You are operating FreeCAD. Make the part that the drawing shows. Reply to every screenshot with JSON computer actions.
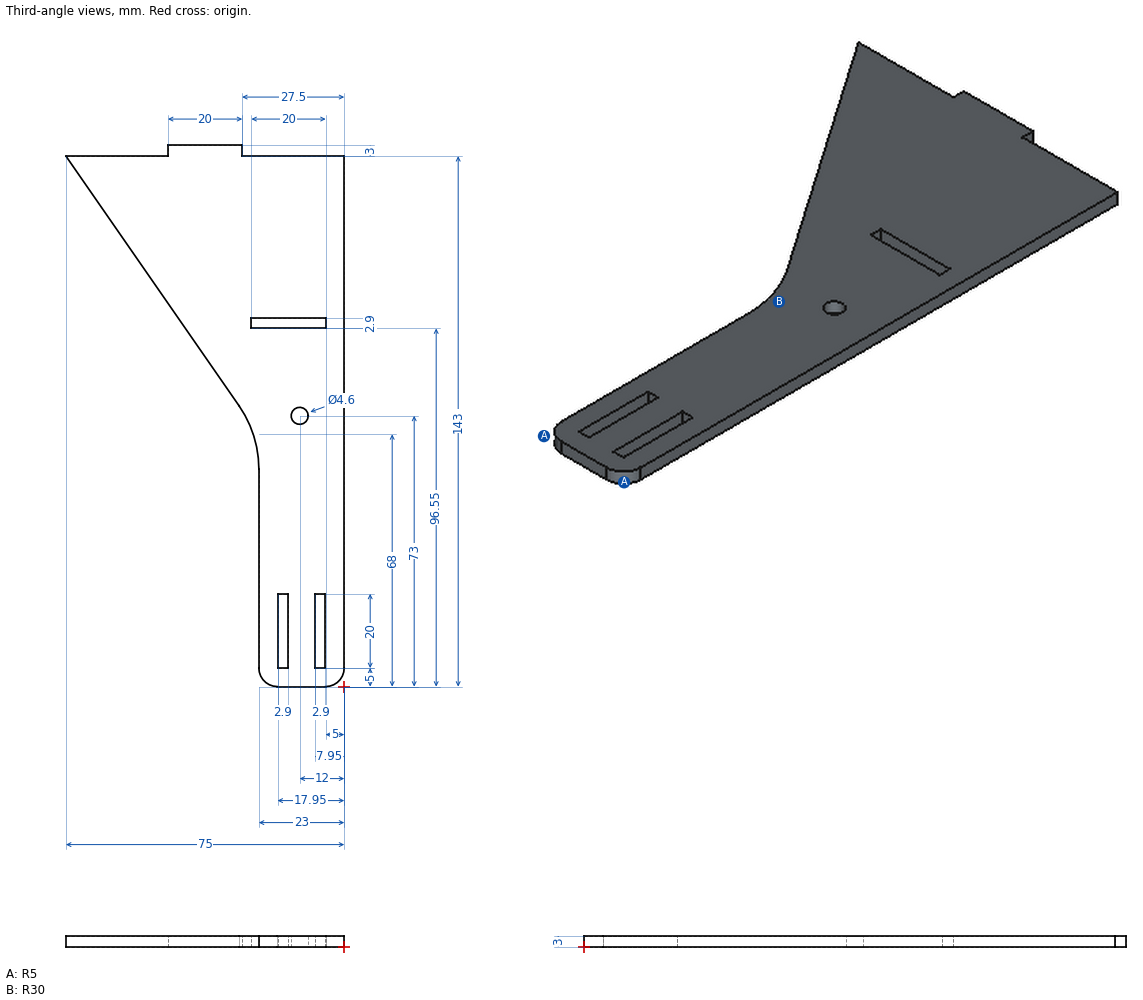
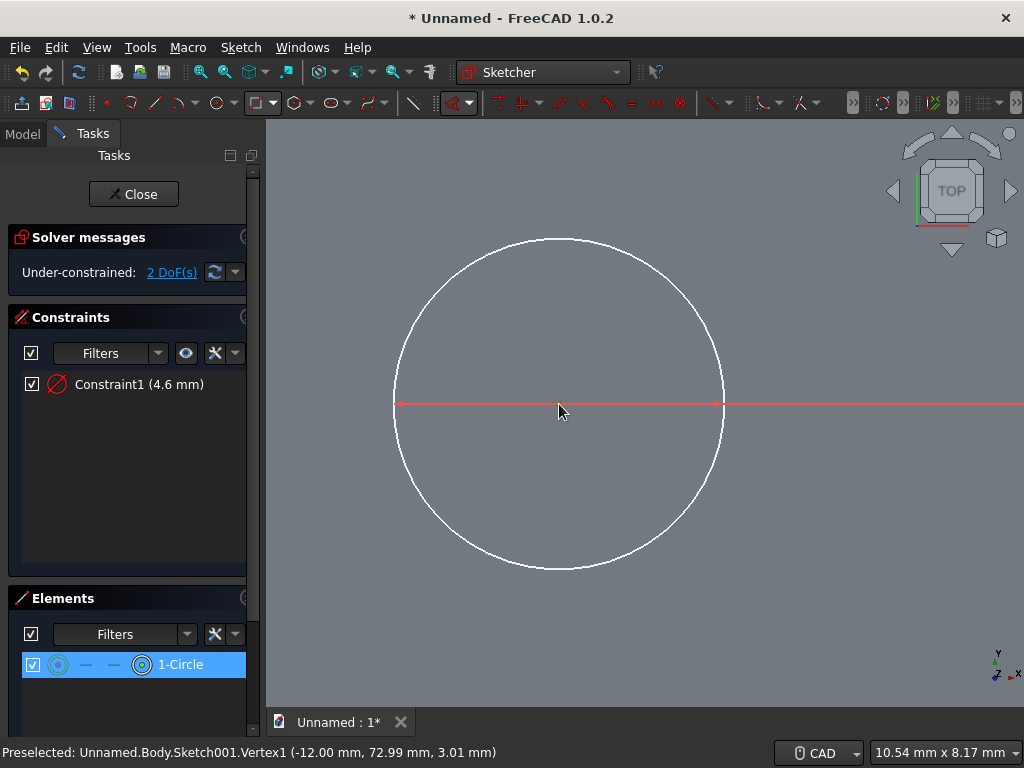
{"action": "left_click", "coordinate": [472, 104]}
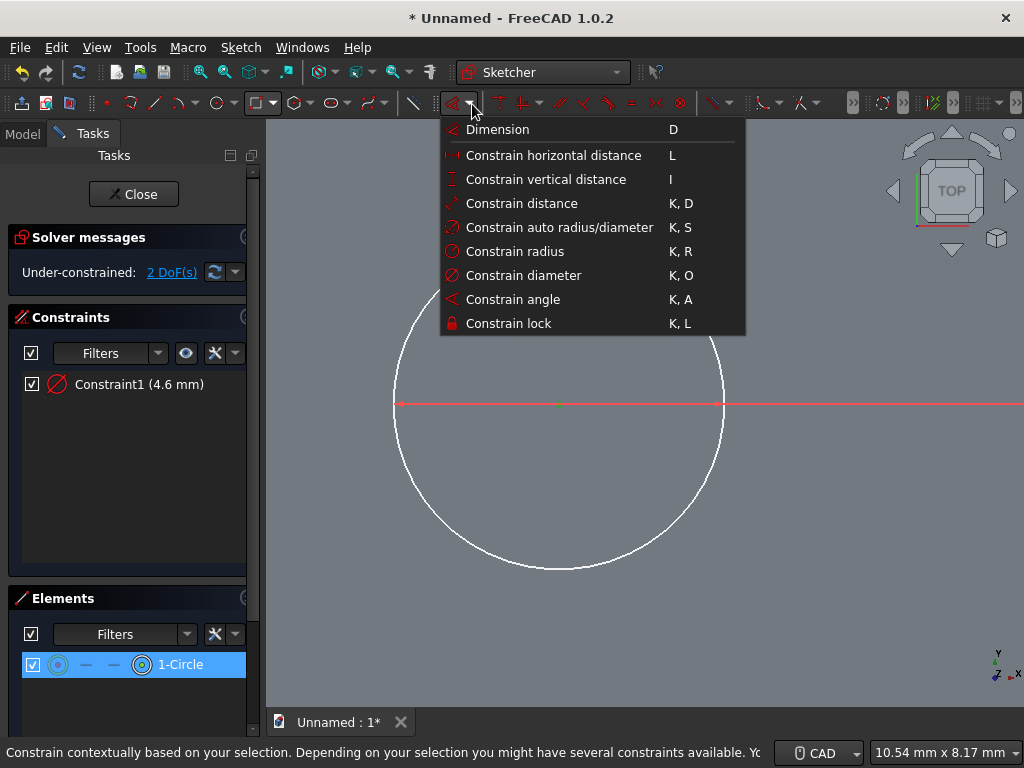
{"action": "left_click", "coordinate": [593, 155]}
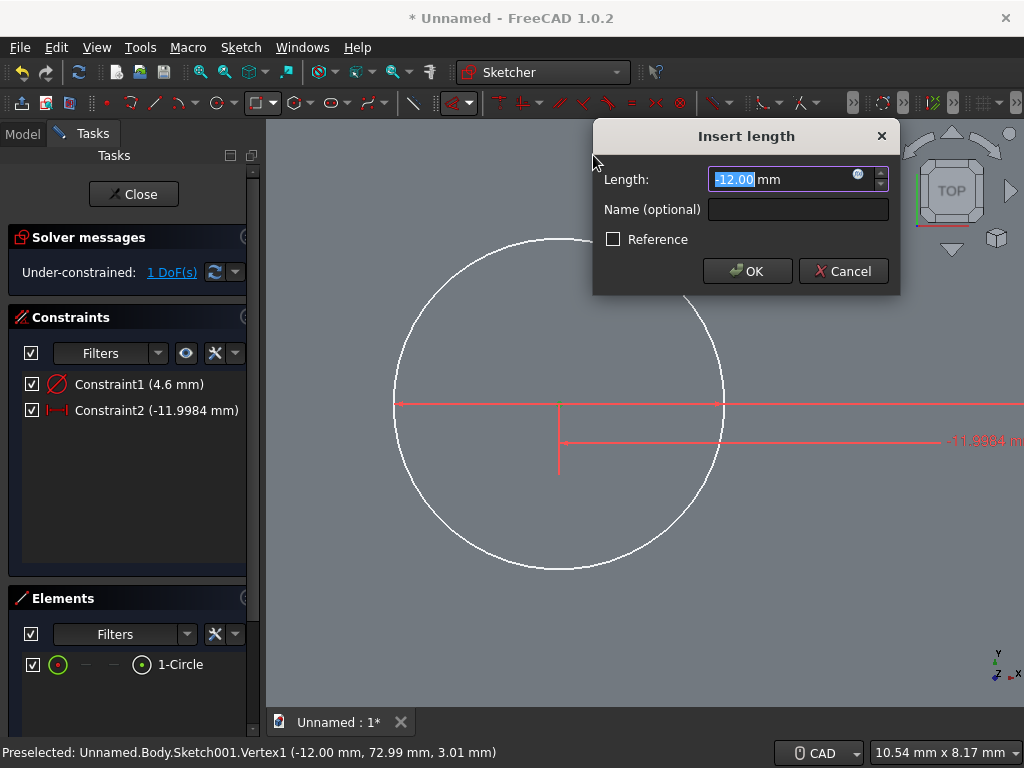
{"action": "type", "text": "-12"}
{"action": "key", "text": "Return"}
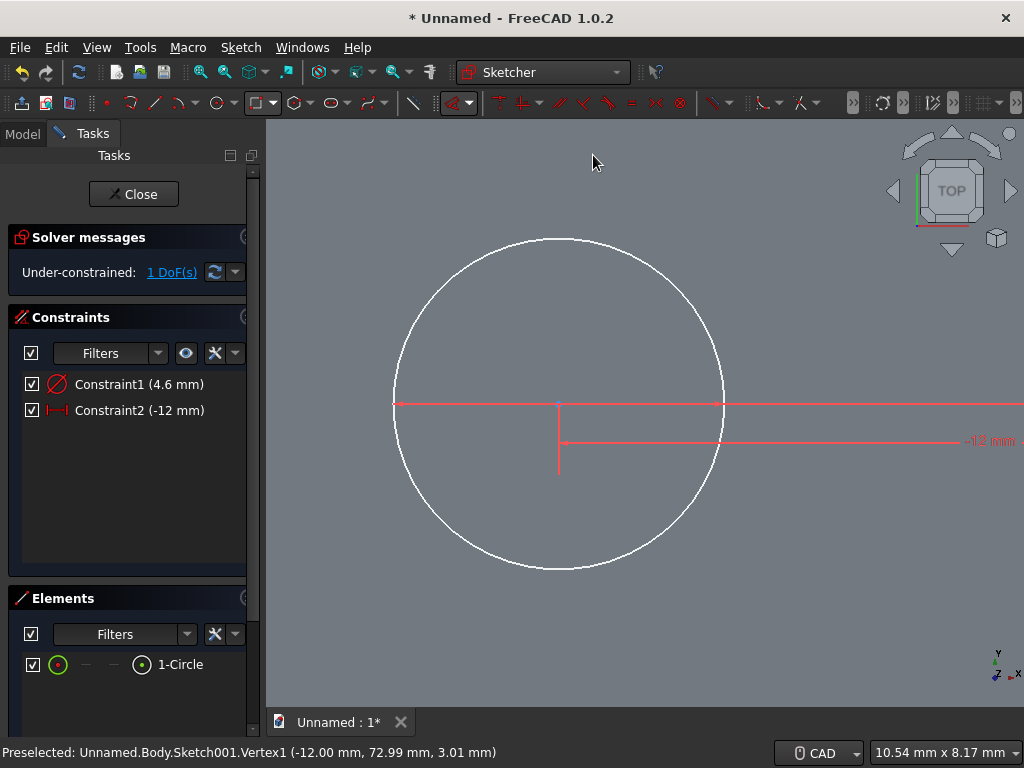
{"action": "left_click", "coordinate": [559, 404]}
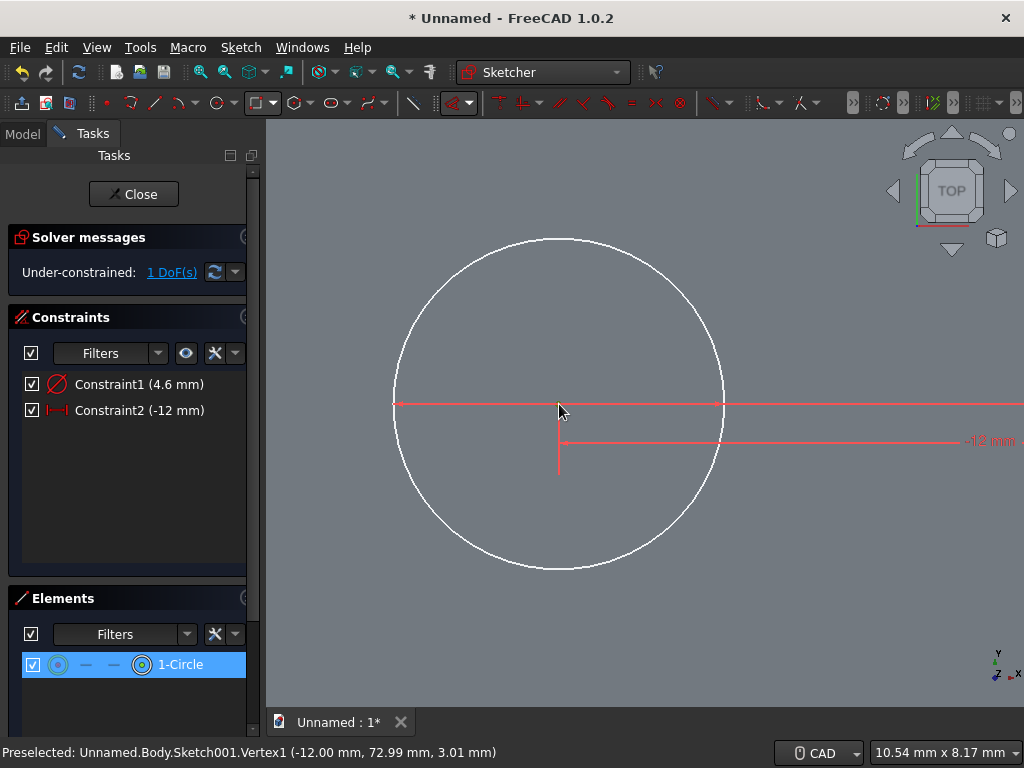
{"action": "key", "text": "i"}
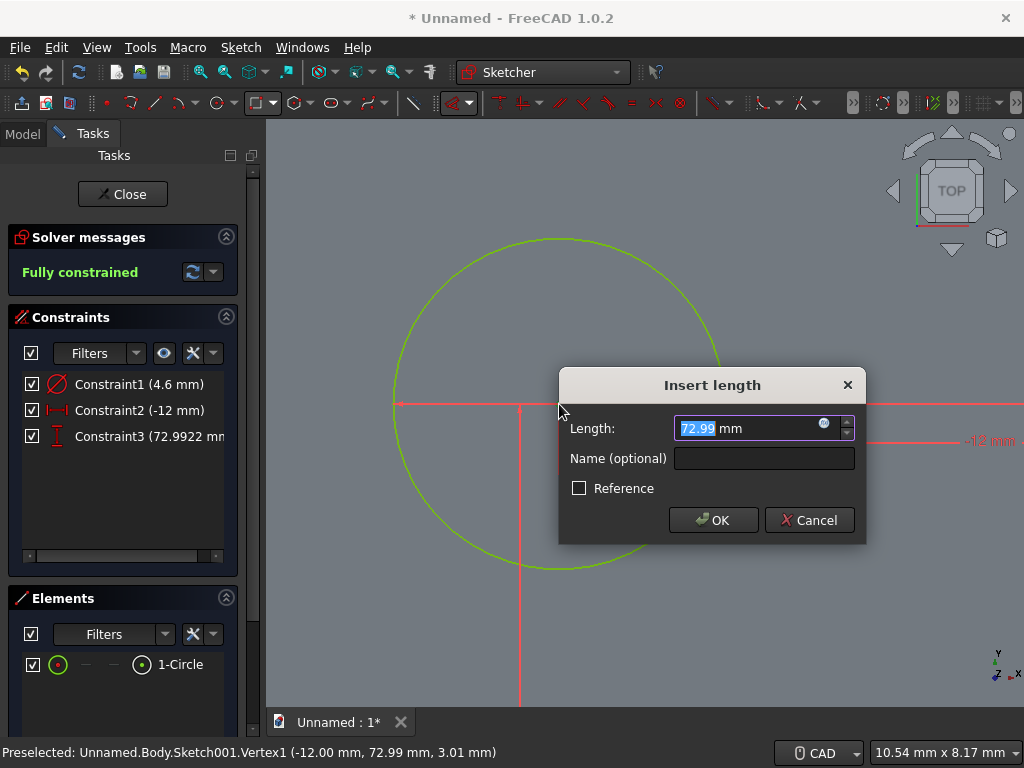
{"action": "type", "text": "73"}
{"action": "key", "text": "Return"}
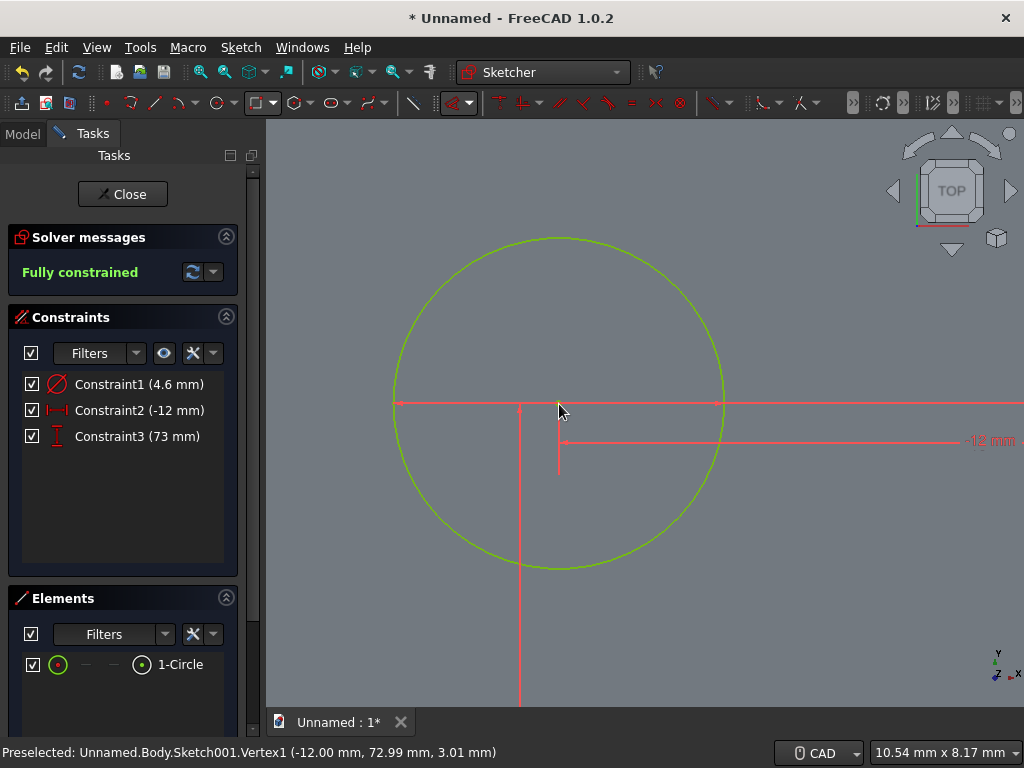
{"action": "left_click", "coordinate": [123, 194]}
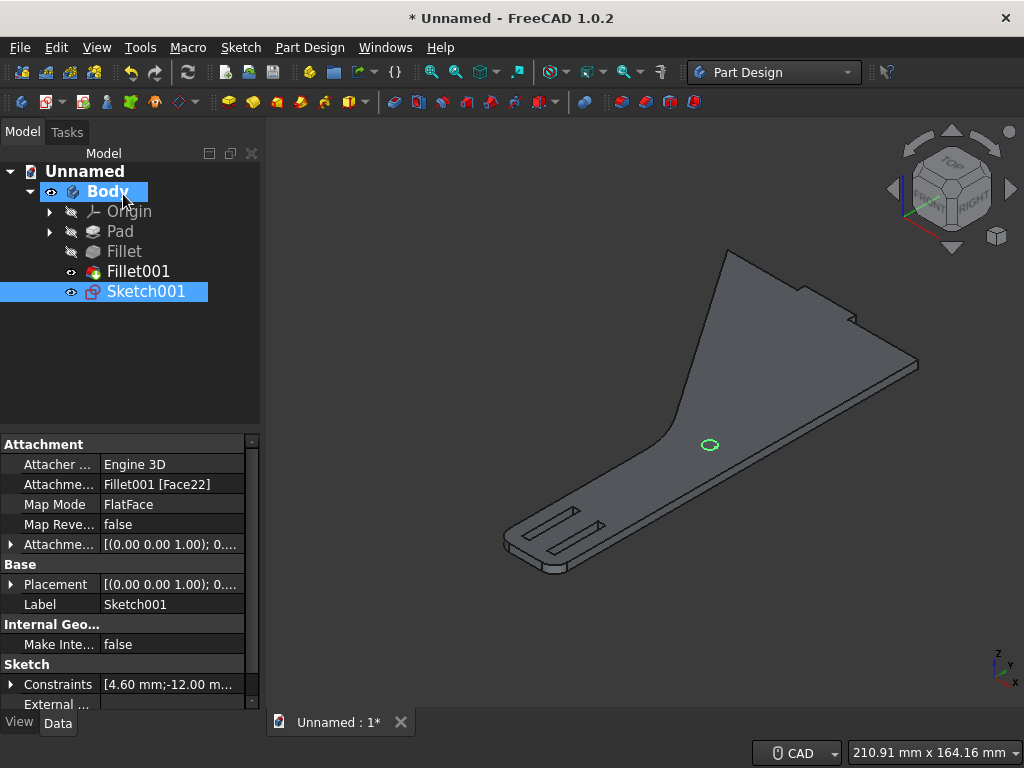
{"action": "left_click", "coordinate": [396, 102]}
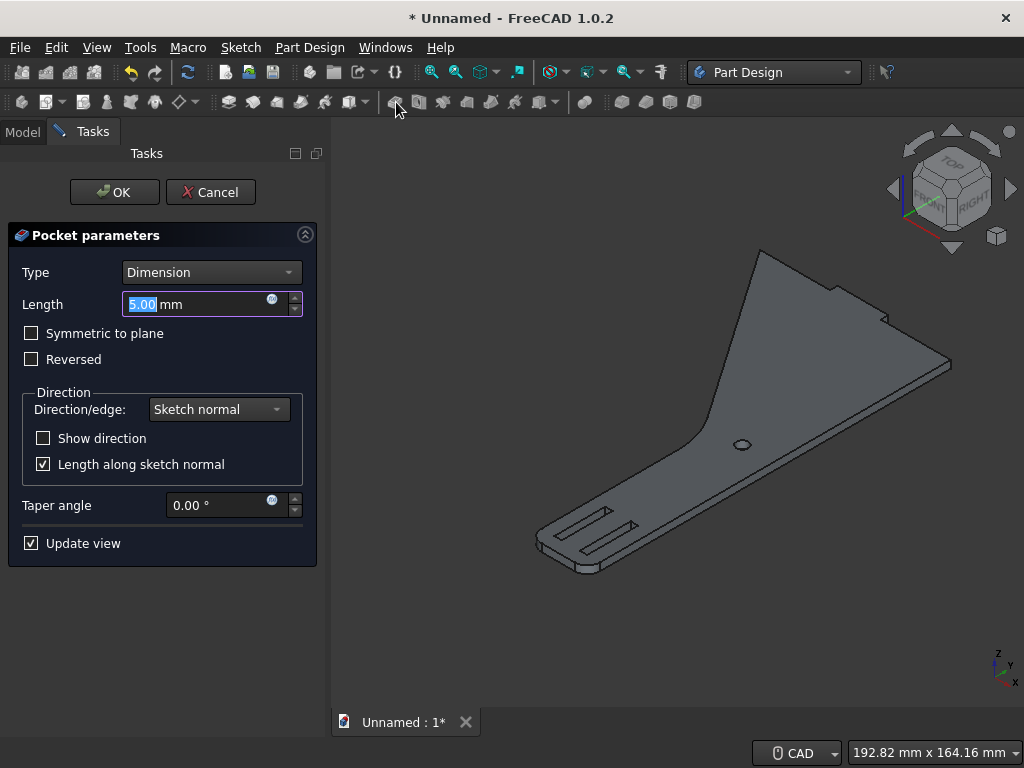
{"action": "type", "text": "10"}
{"action": "key", "text": "Tab"}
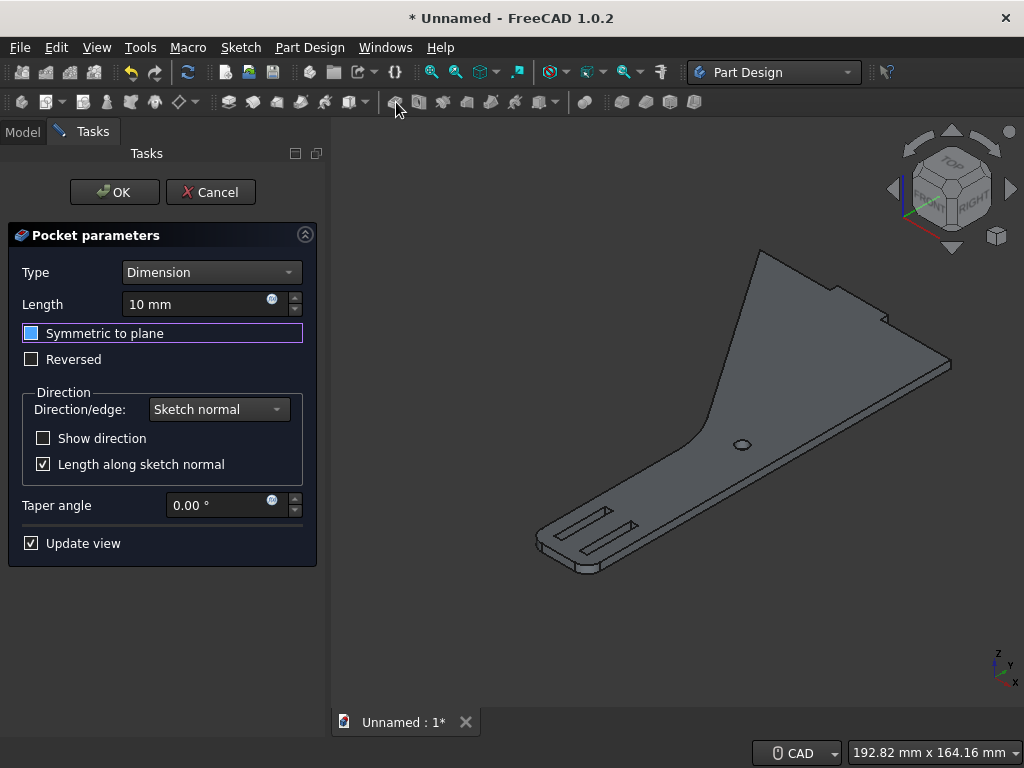
{"action": "left_click", "coordinate": [115, 192]}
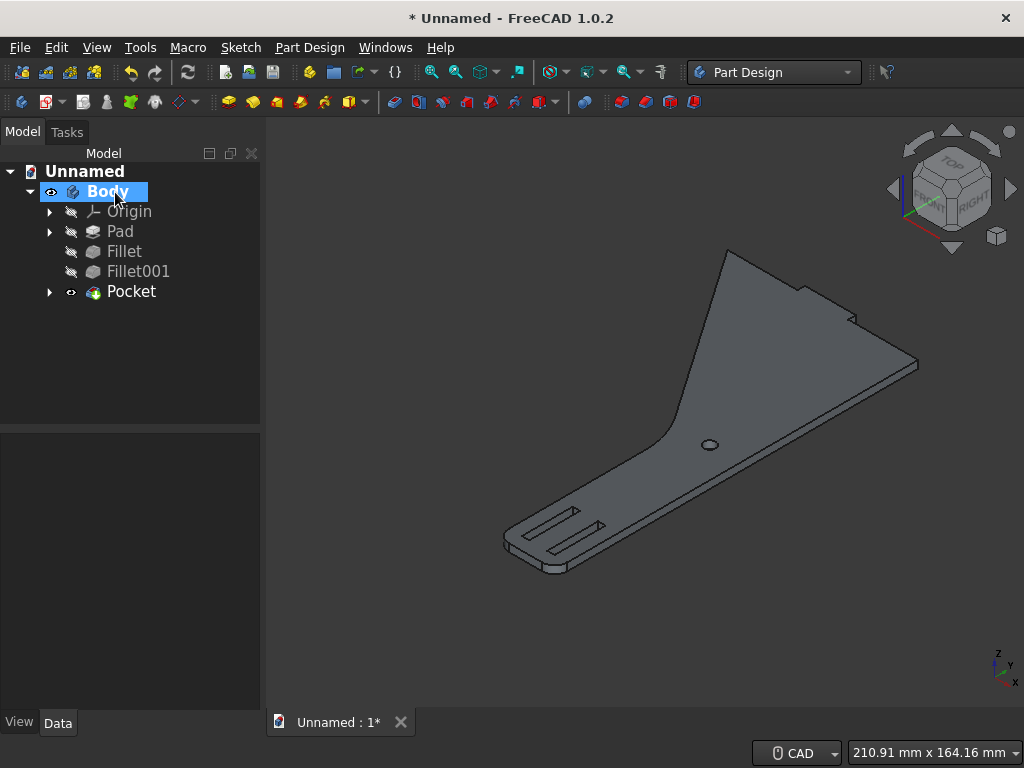
{"action": "key", "text": "5"}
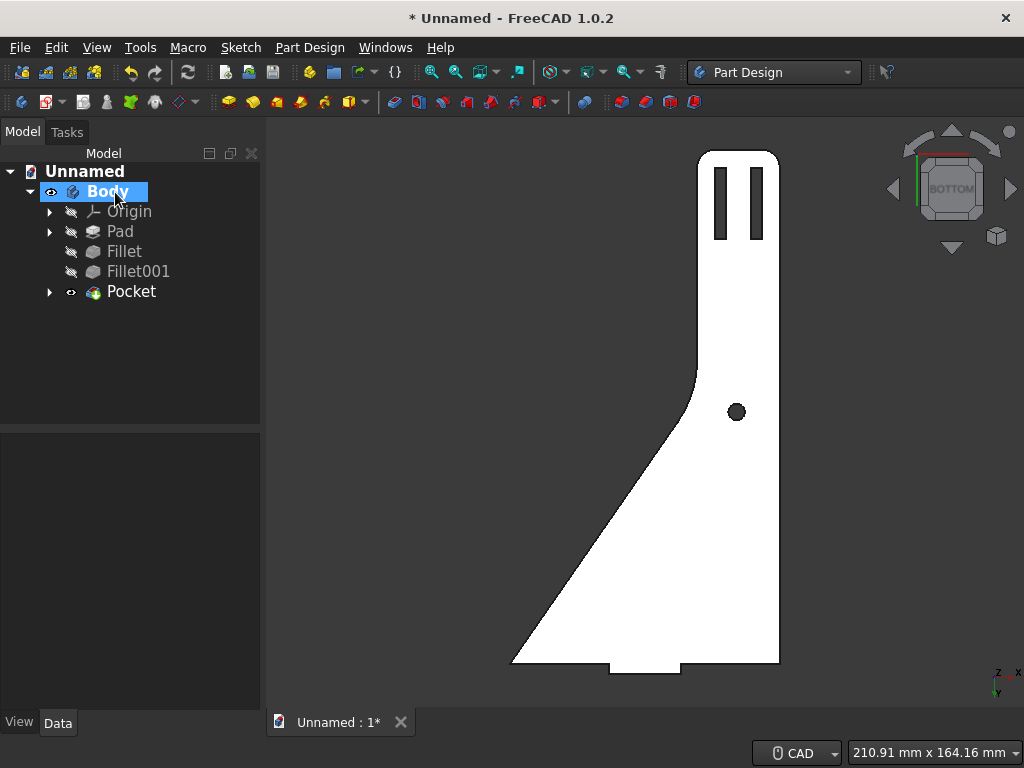
{"action": "left_click", "coordinate": [684, 561]}